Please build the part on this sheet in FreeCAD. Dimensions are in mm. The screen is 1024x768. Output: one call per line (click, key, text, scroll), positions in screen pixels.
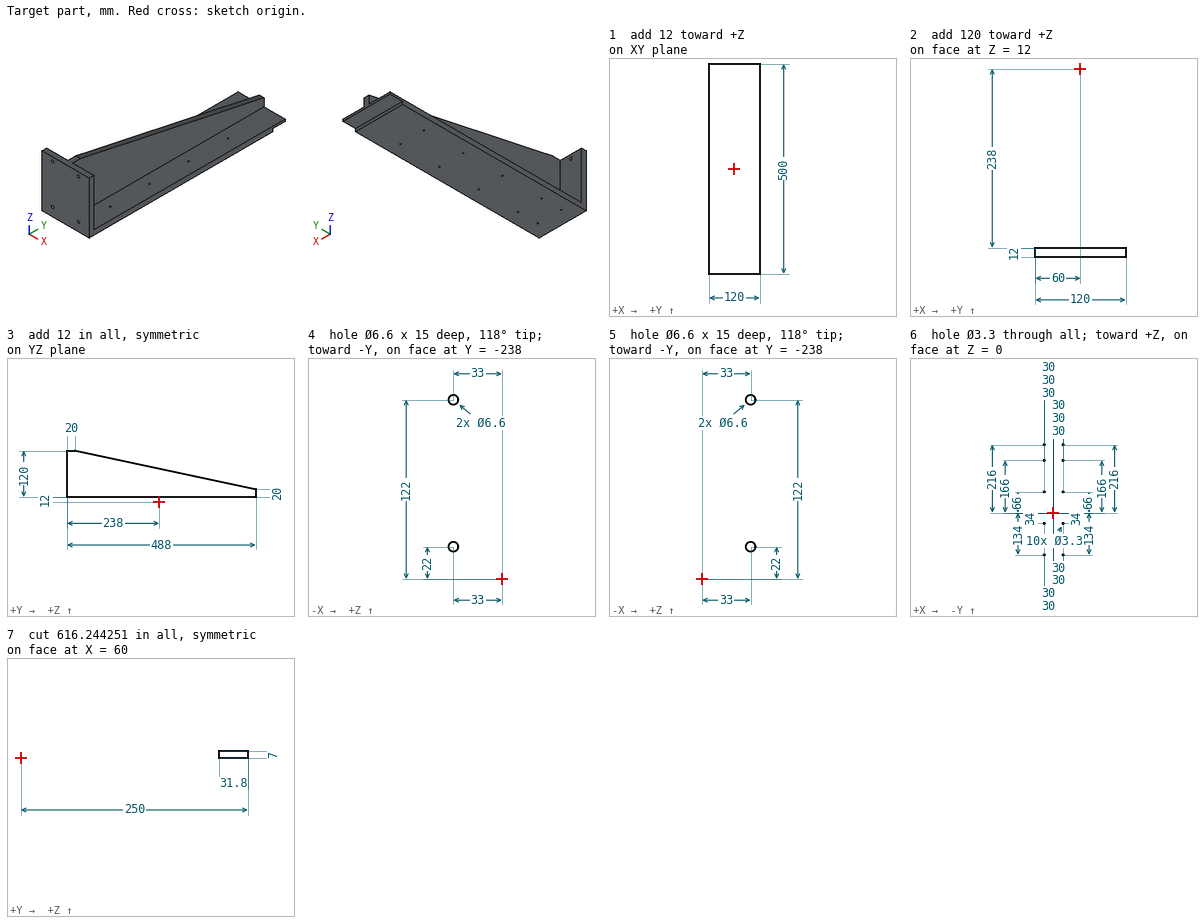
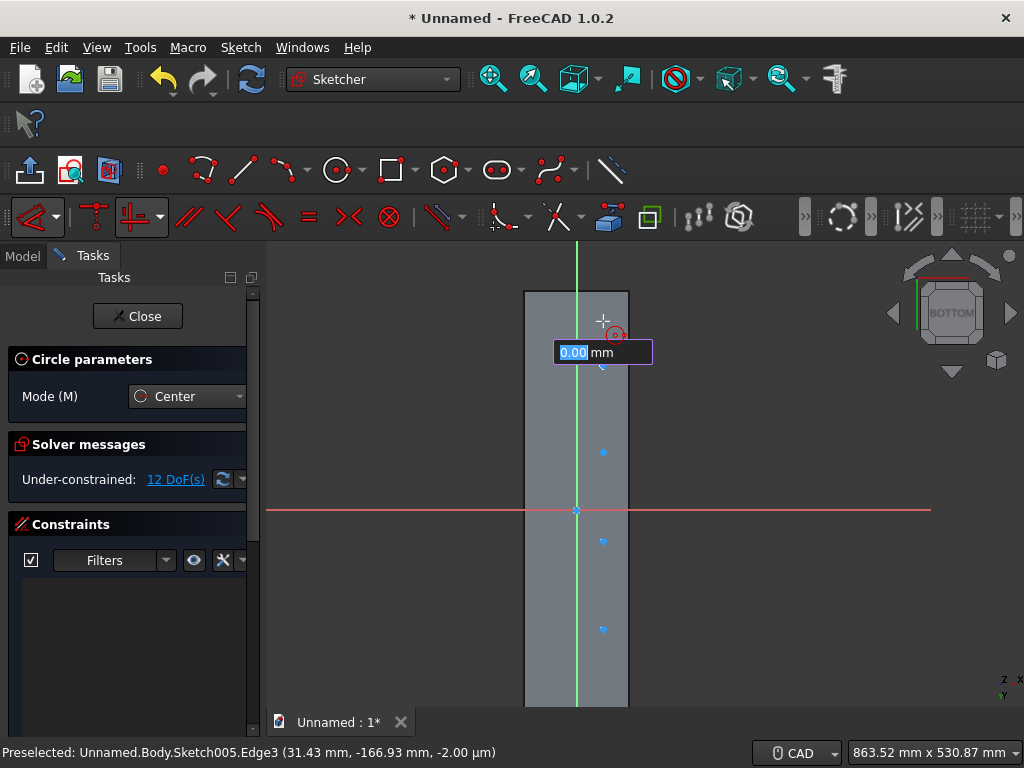
scroll(604, 320, up, 12)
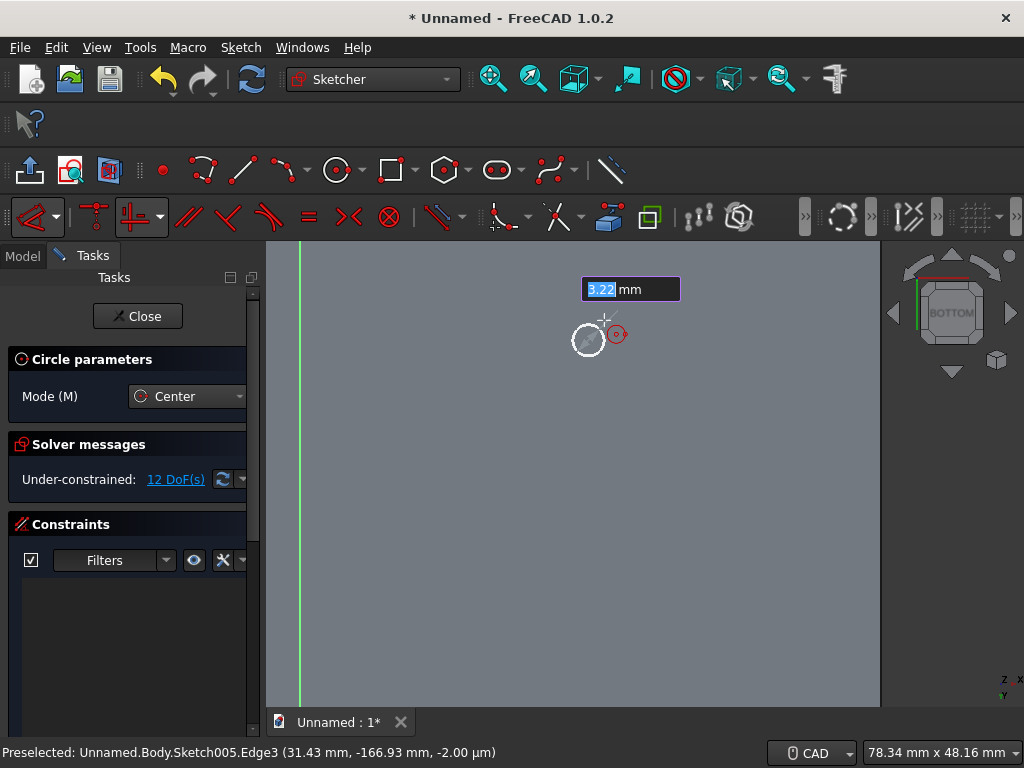
click(602, 315)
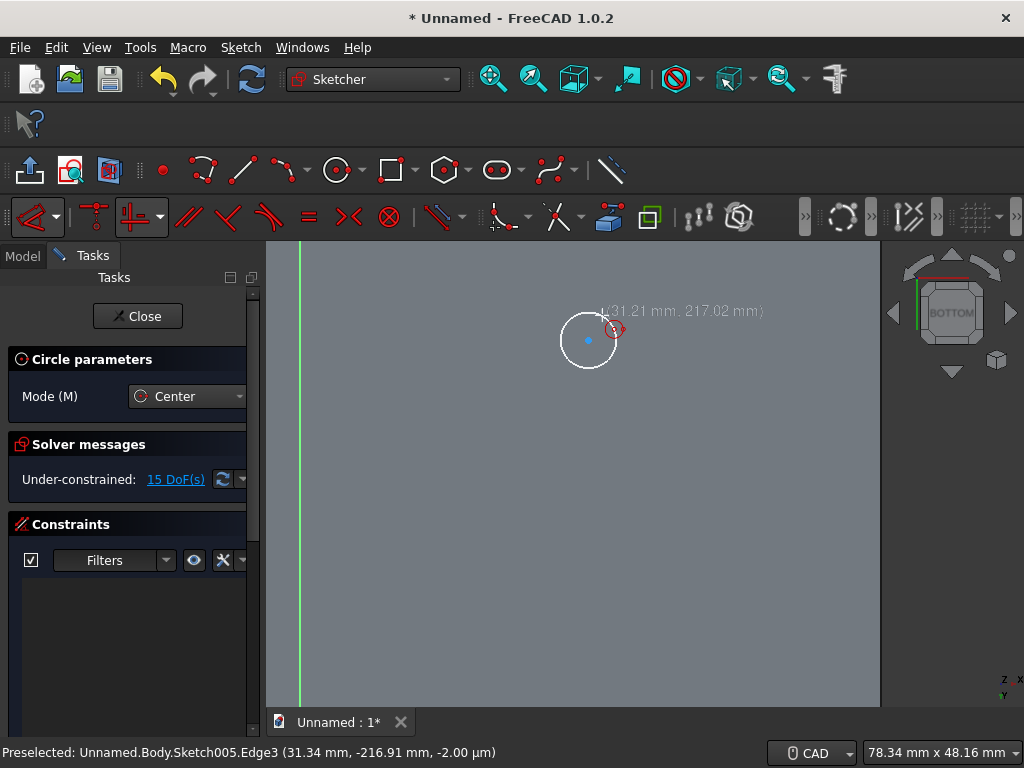
scroll(604, 320, down, 12)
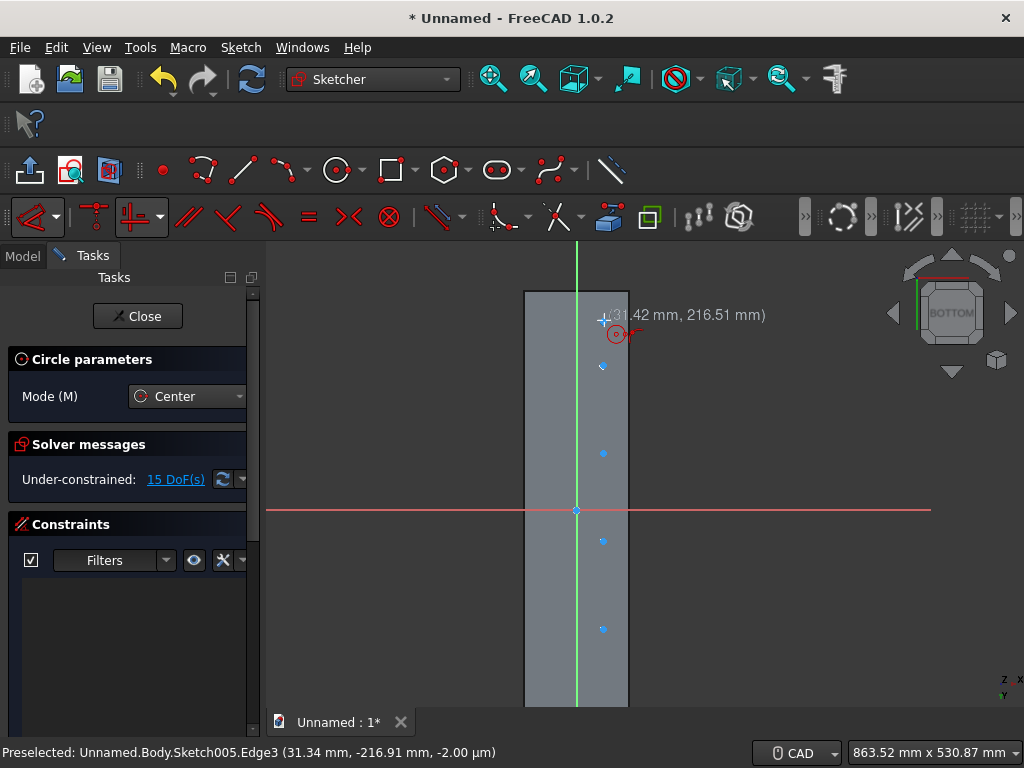
scroll(550, 321, up, 14)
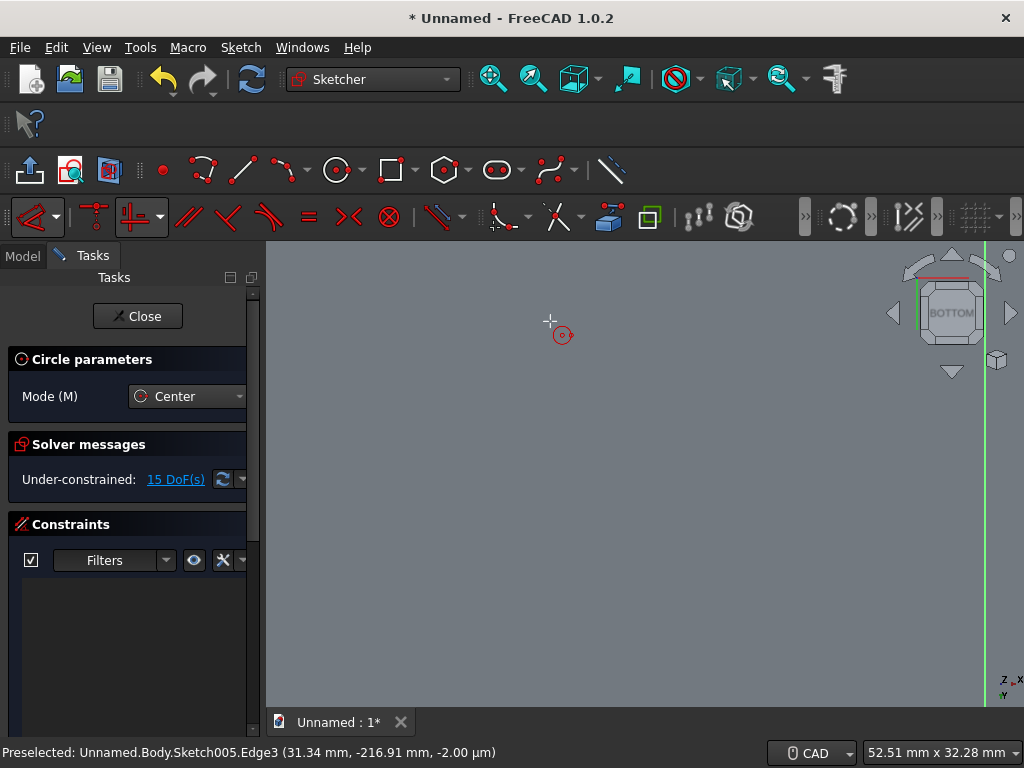
scroll(550, 321, down, 14)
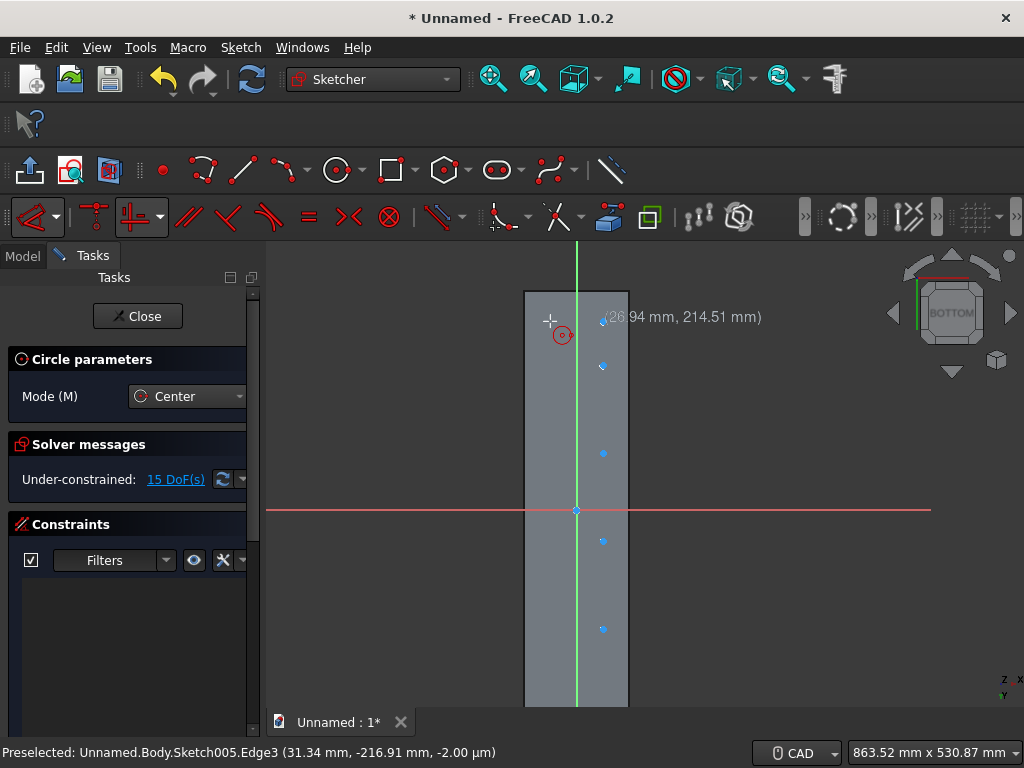
click(550, 321)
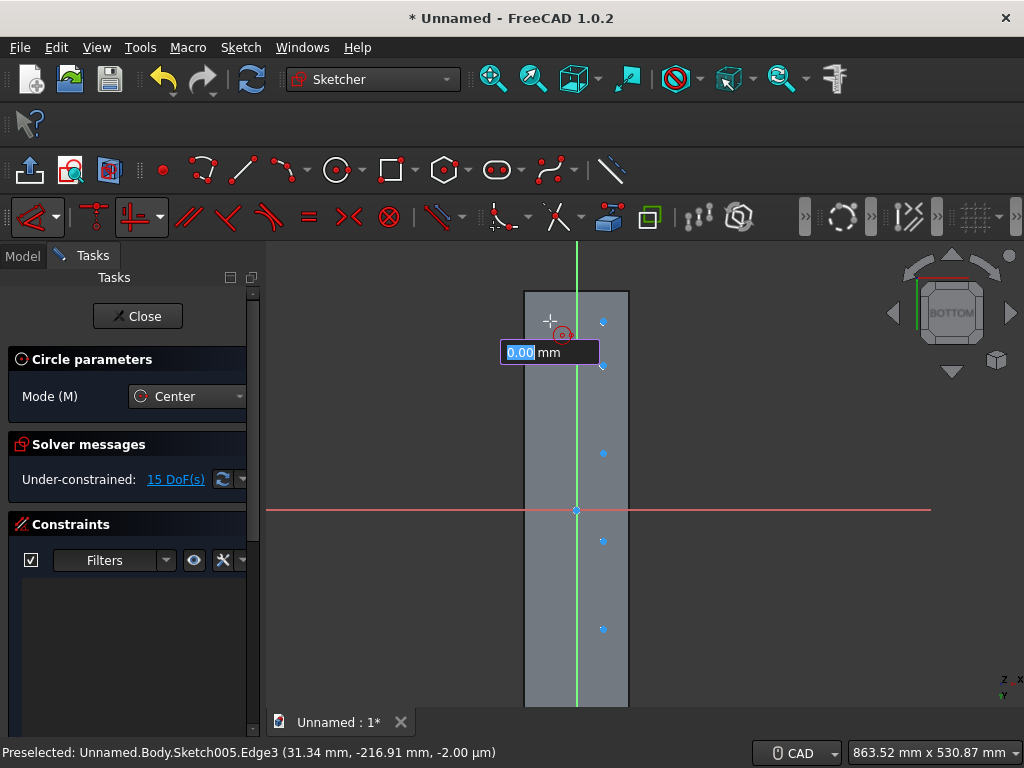
scroll(552, 320, up, 12)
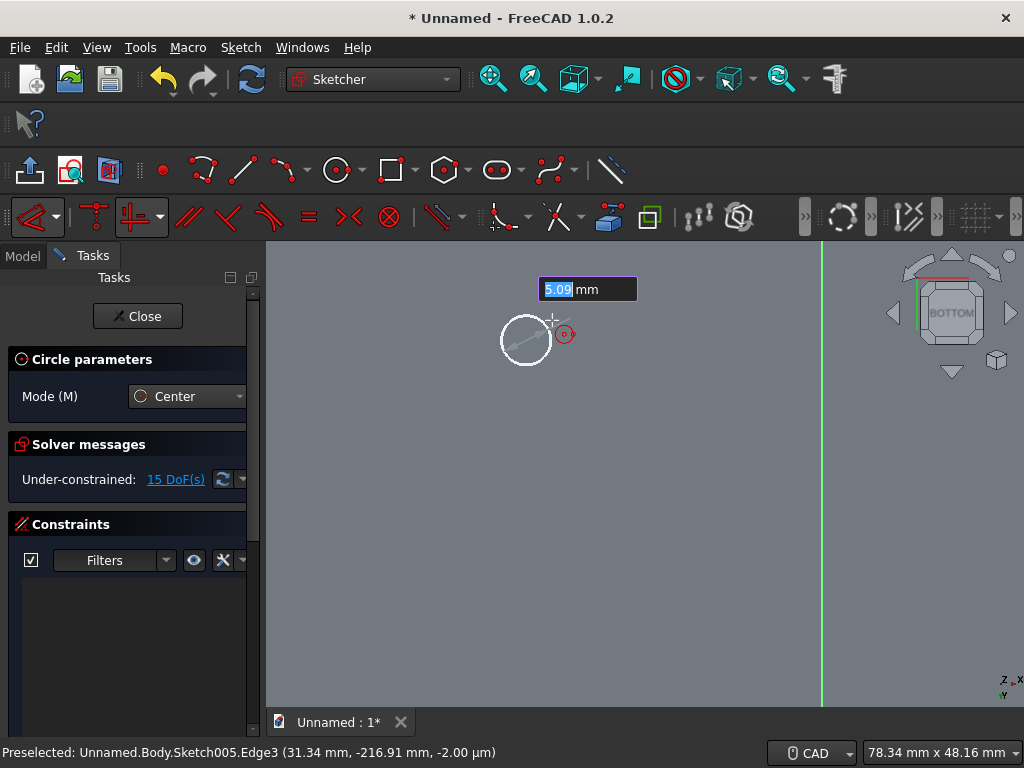
click(543, 315)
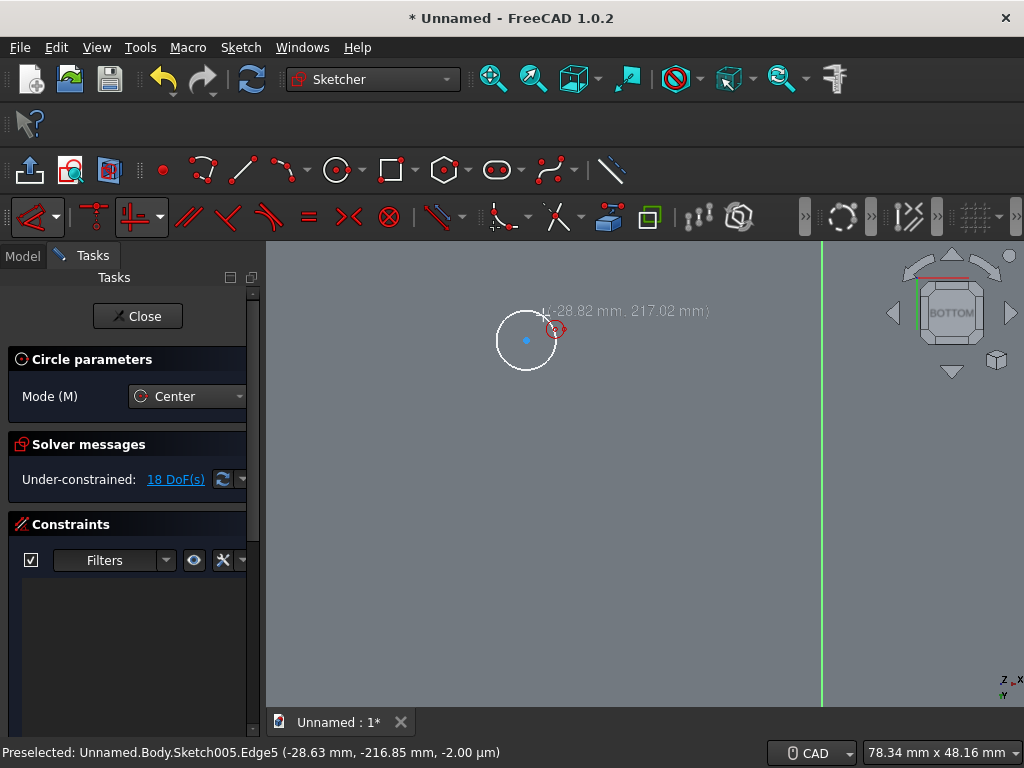
scroll(552, 320, down, 12)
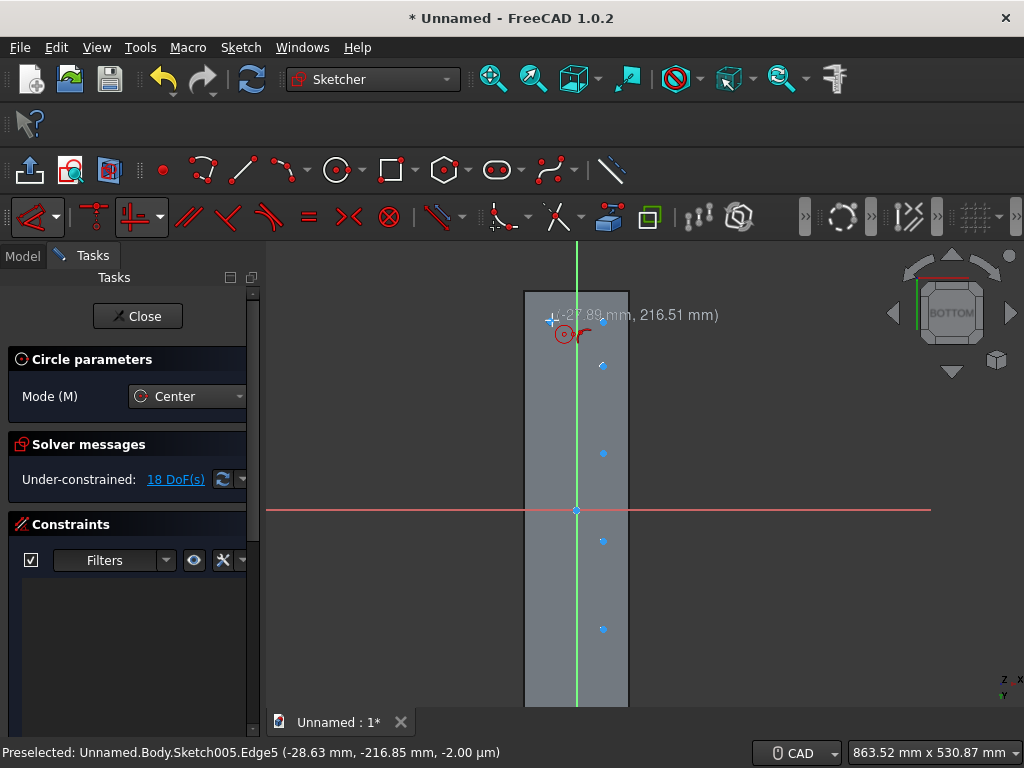
scroll(550, 365, up, 14)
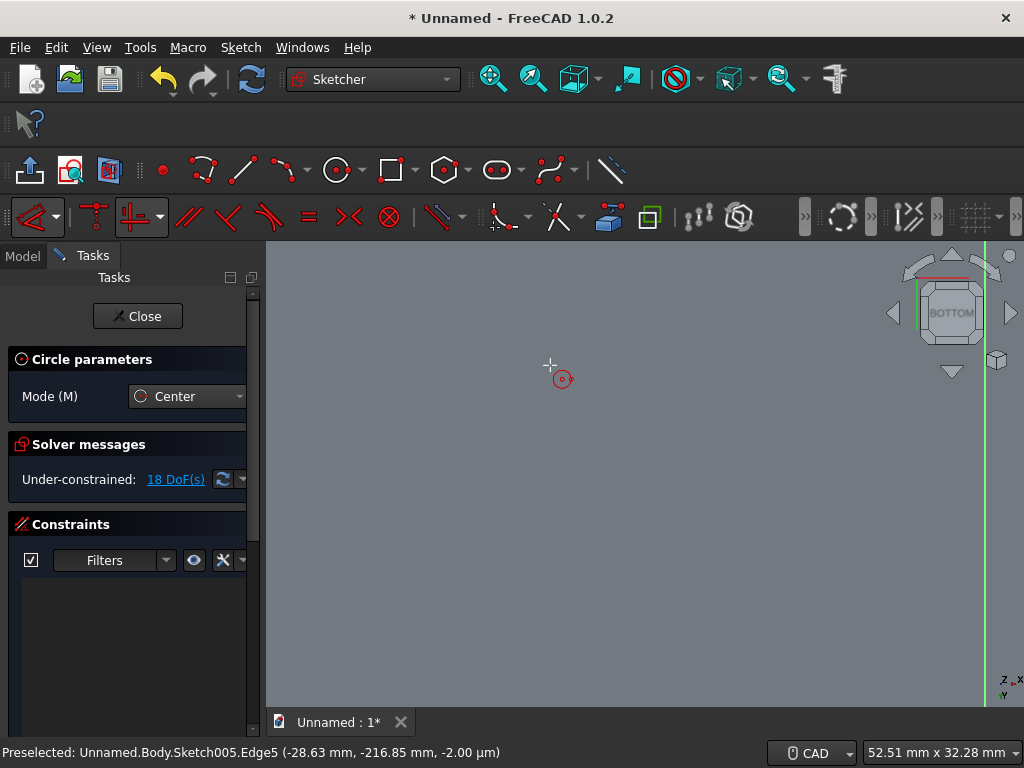
scroll(550, 365, down, 14)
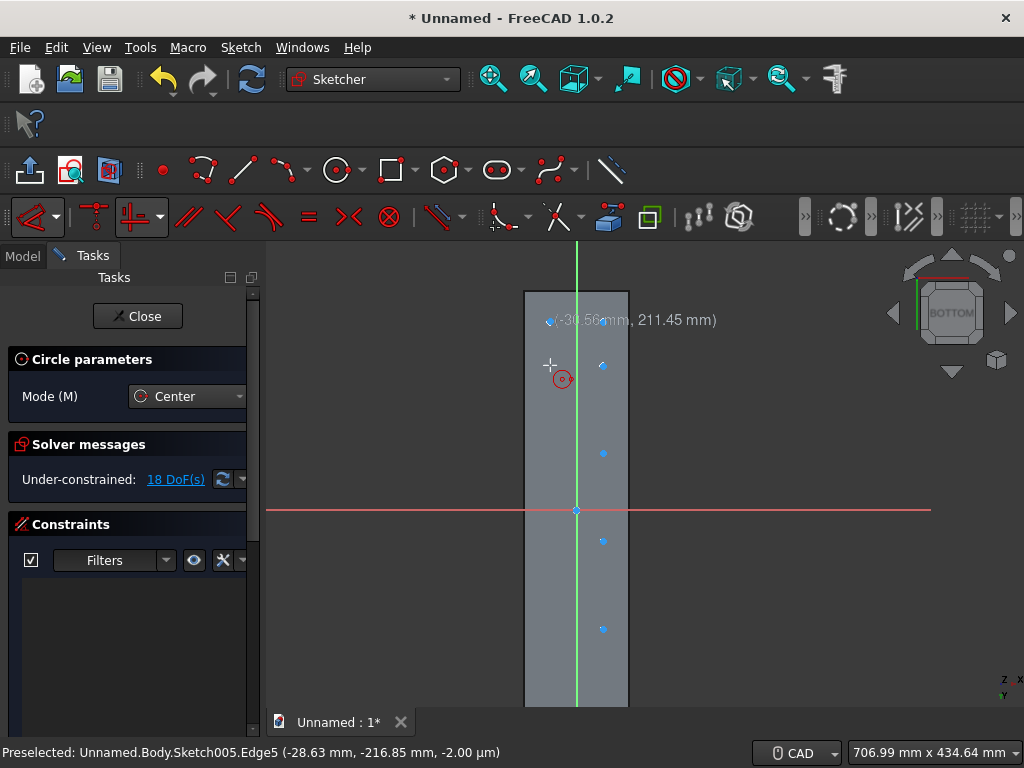
click(550, 365)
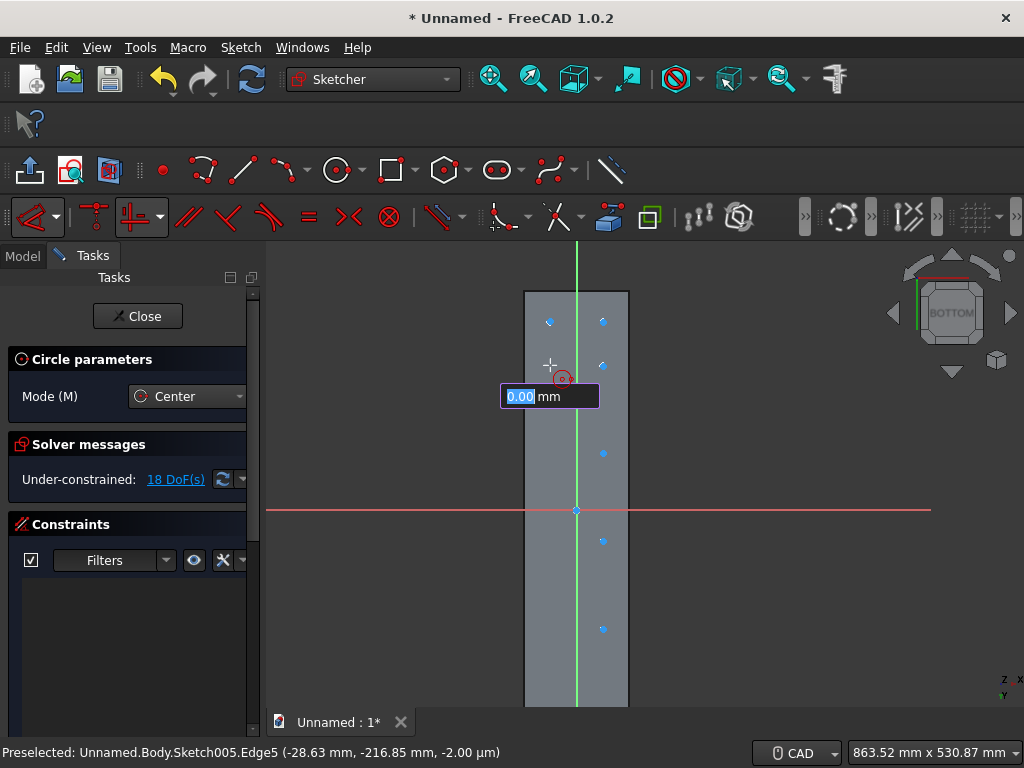
scroll(552, 364, up, 12)